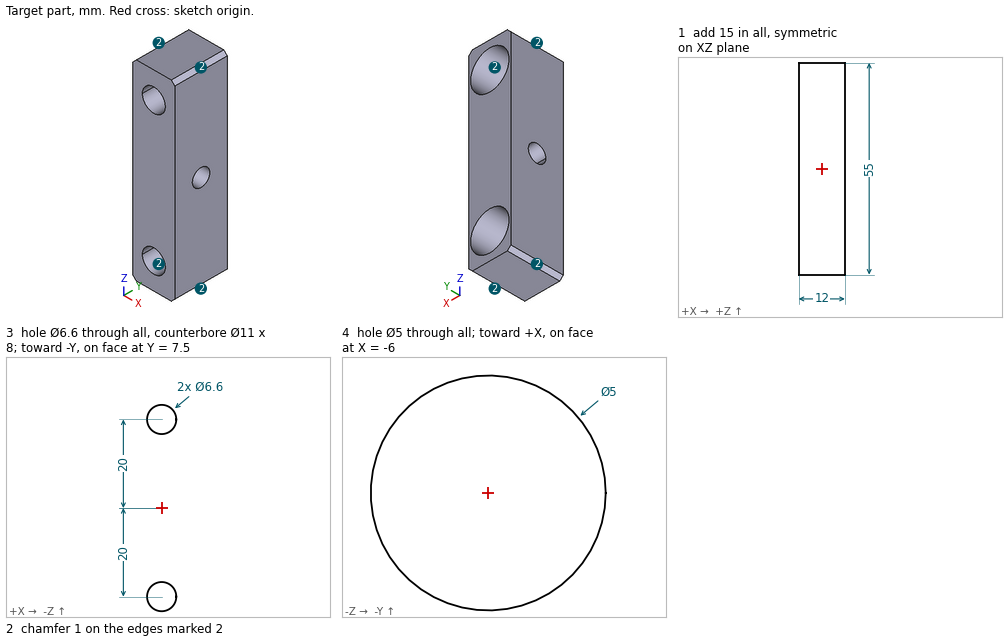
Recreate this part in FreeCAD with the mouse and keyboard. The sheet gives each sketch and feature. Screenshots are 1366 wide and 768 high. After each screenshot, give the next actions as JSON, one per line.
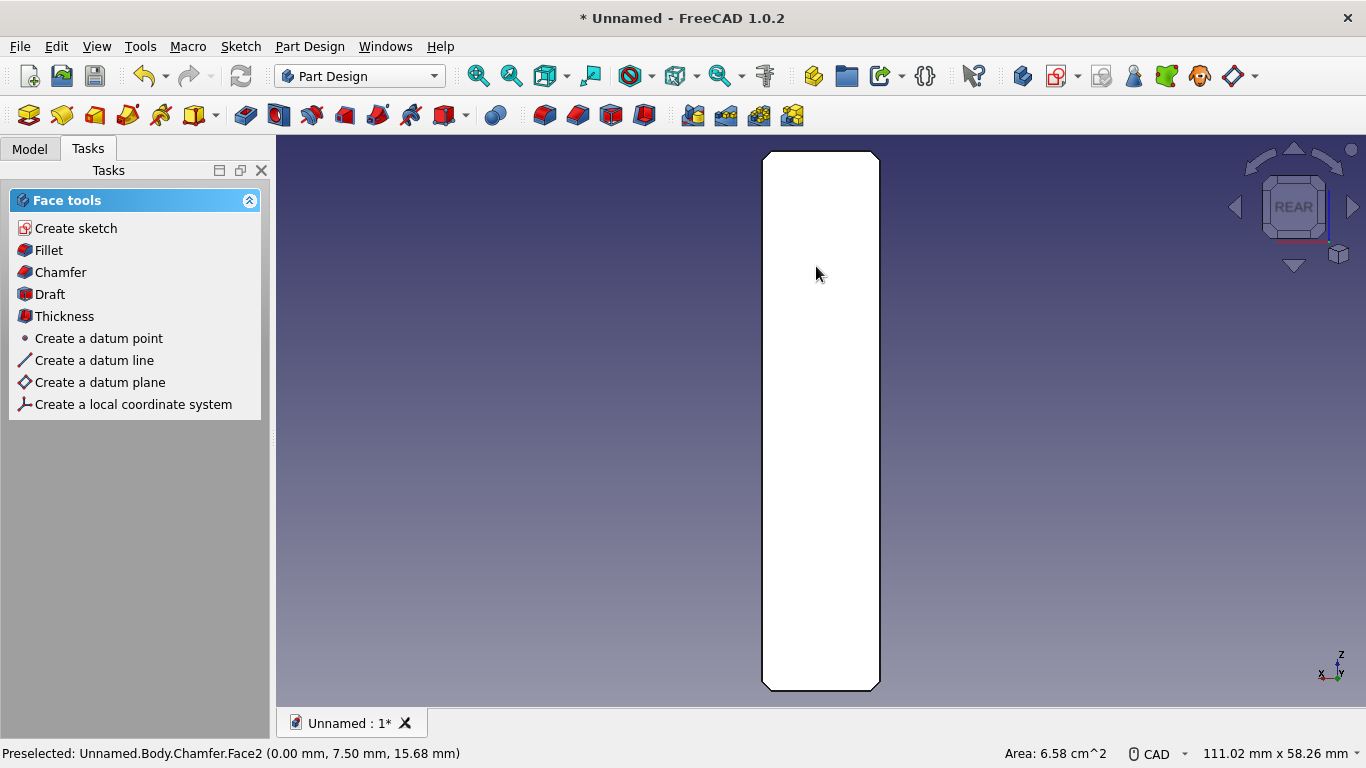
{"action": "left_click", "coordinate": [1056, 76]}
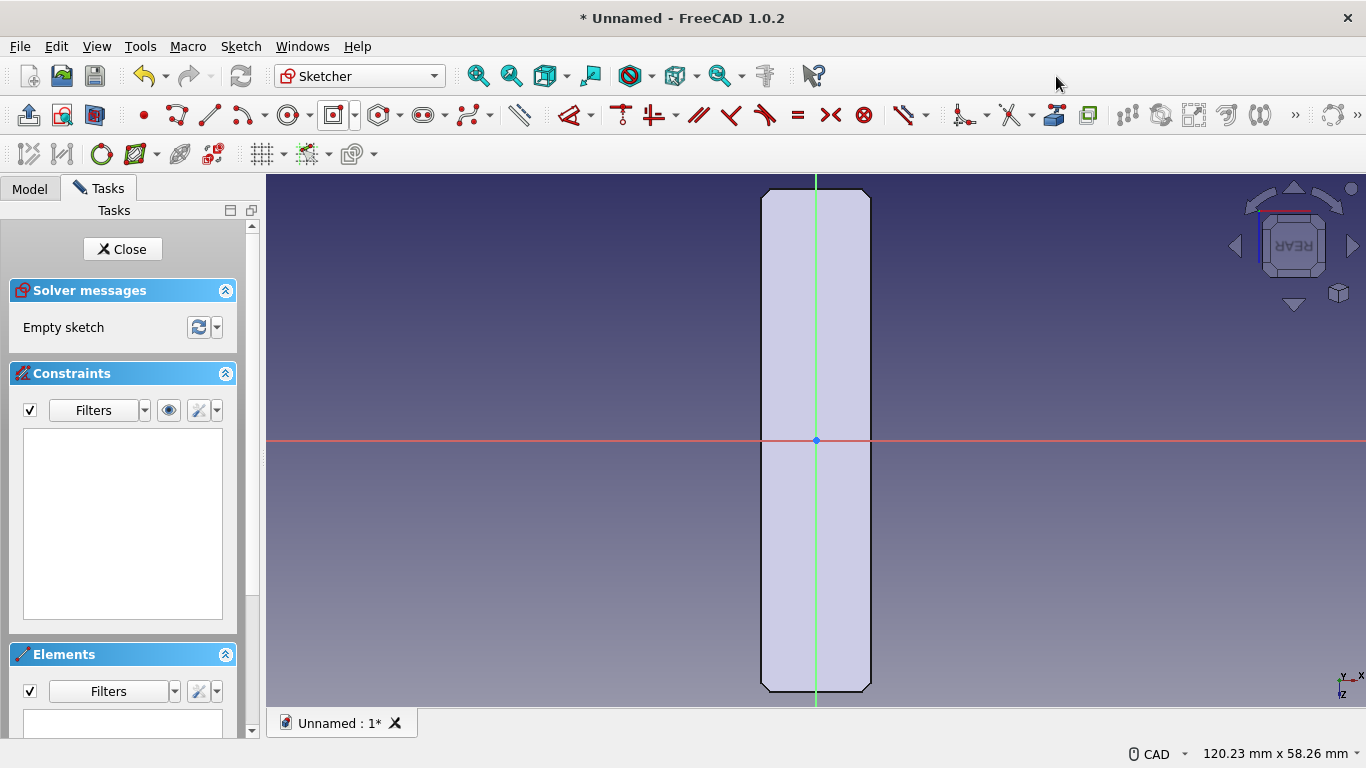
{"action": "left_click", "coordinate": [288, 116]}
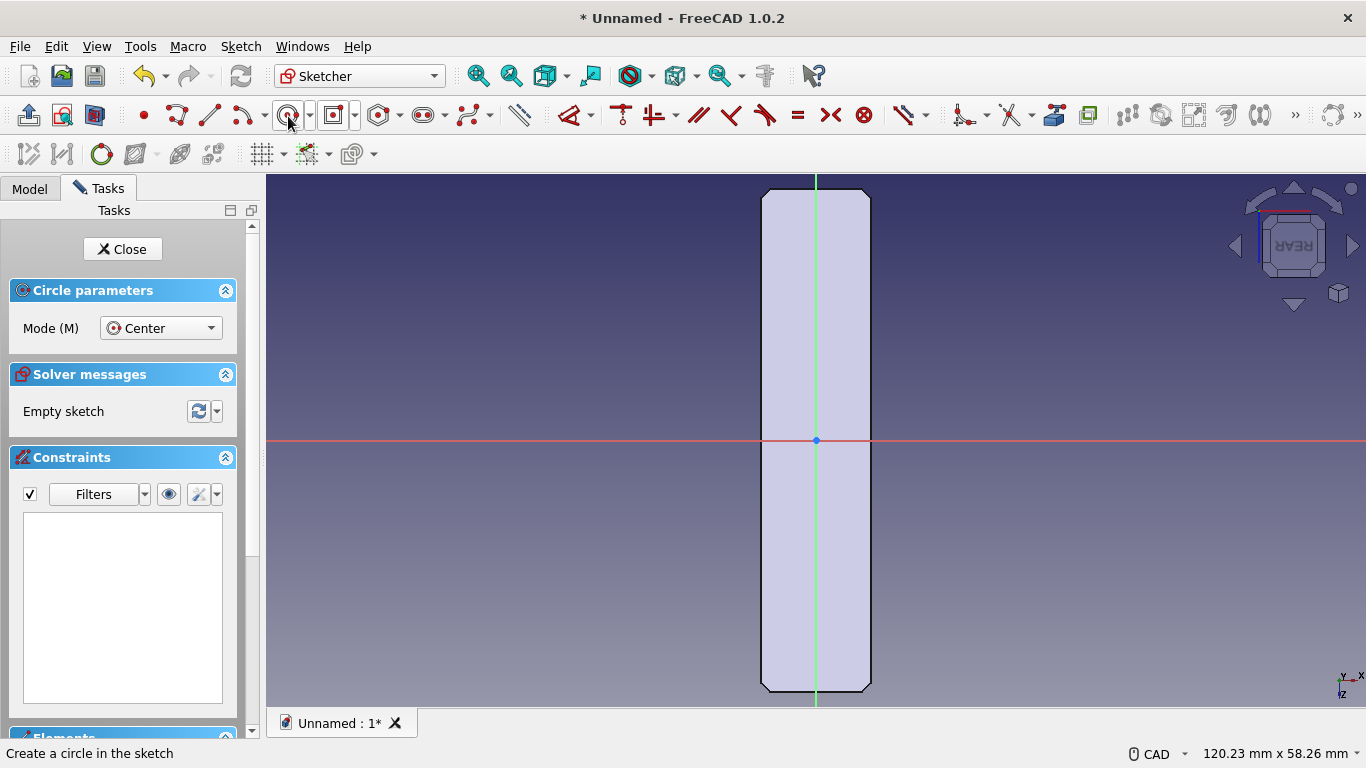
{"action": "left_click", "coordinate": [816, 258]}
{"action": "mouse_move", "coordinate": [837, 236]}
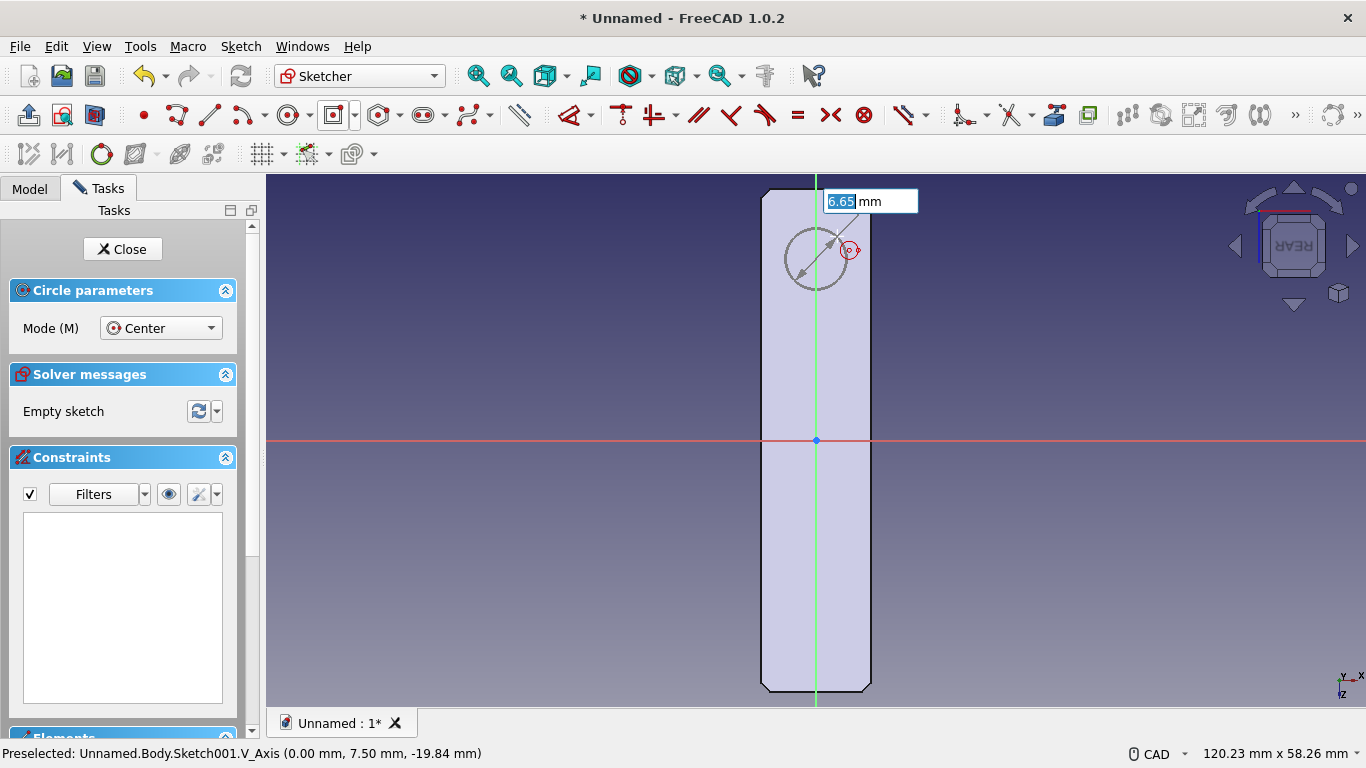
{"action": "type", "text": "6.6"}
{"action": "key", "text": "Return"}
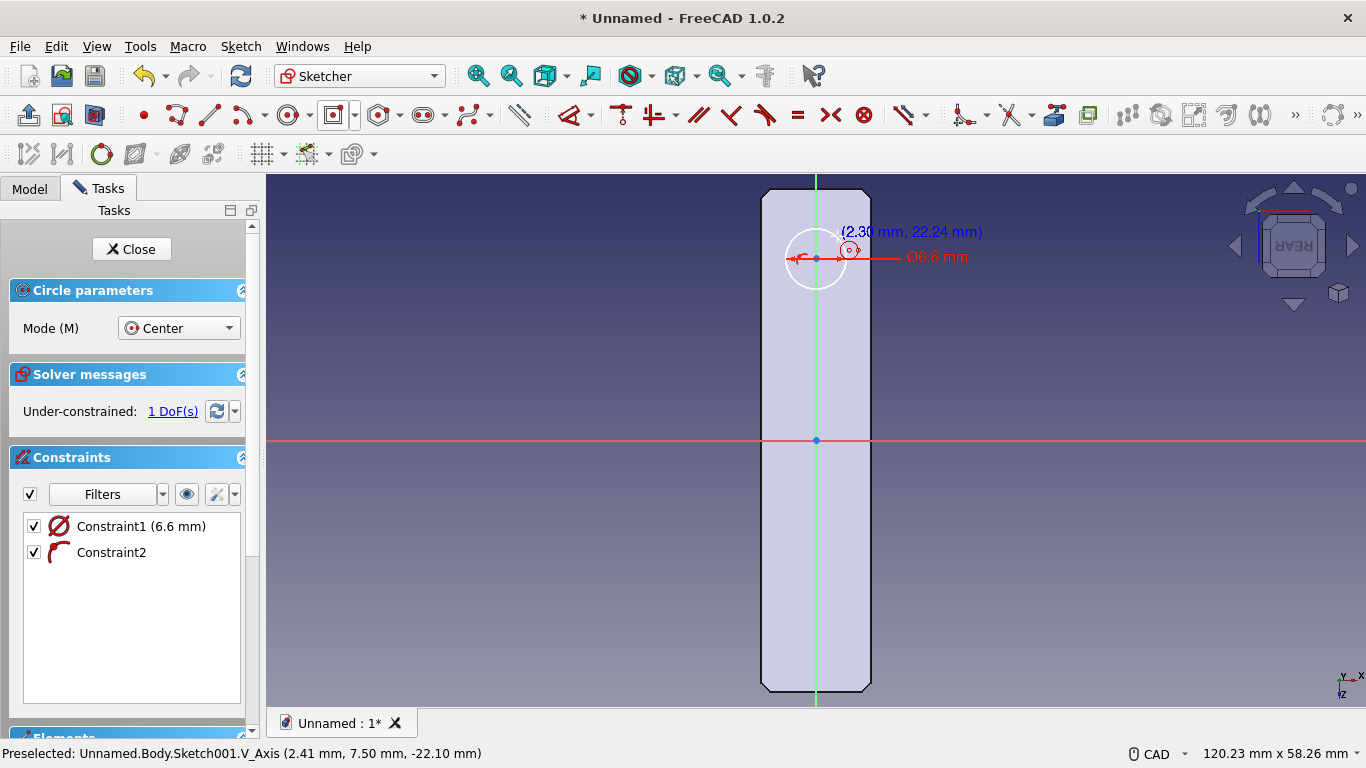
{"action": "left_click", "coordinate": [816, 623]}
{"action": "mouse_move", "coordinate": [837, 602]}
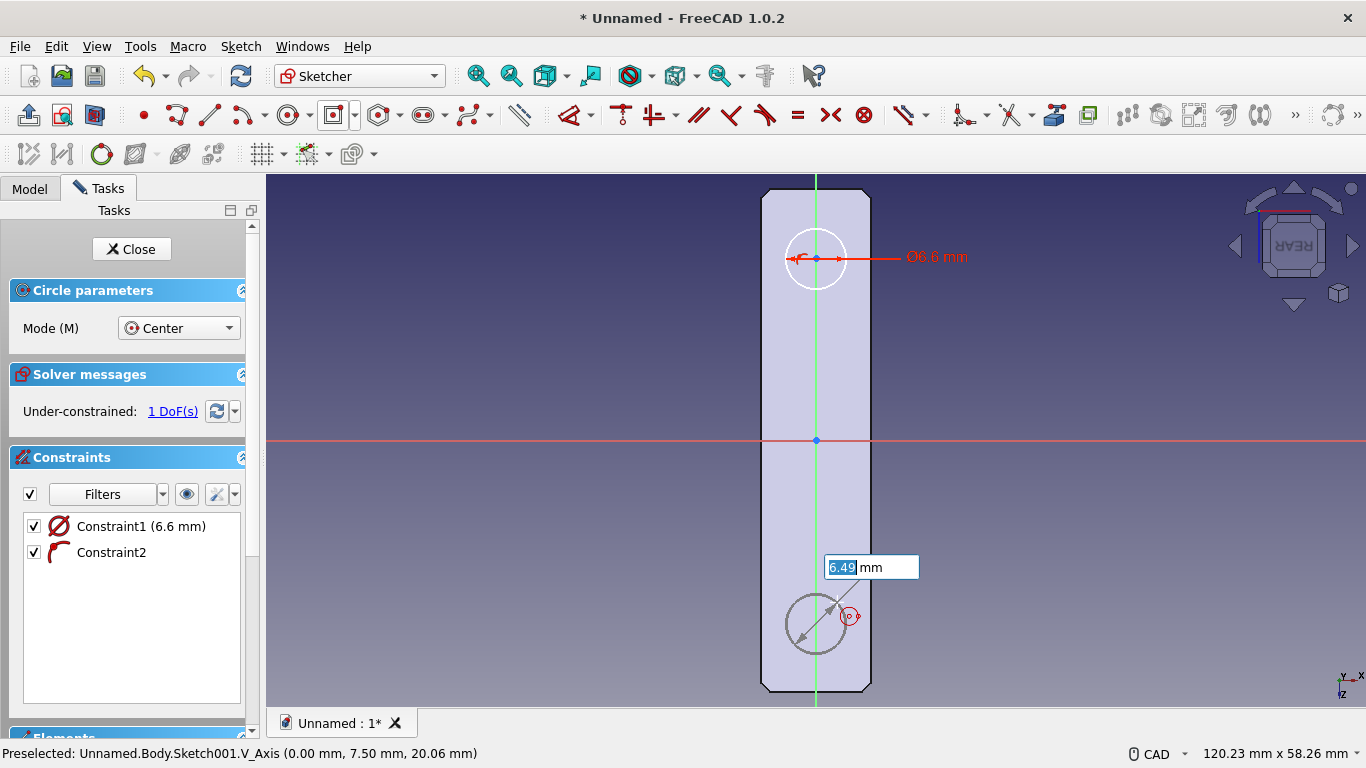
{"action": "type", "text": "6.6"}
{"action": "key", "text": "Return"}
{"action": "key", "text": "Escape"}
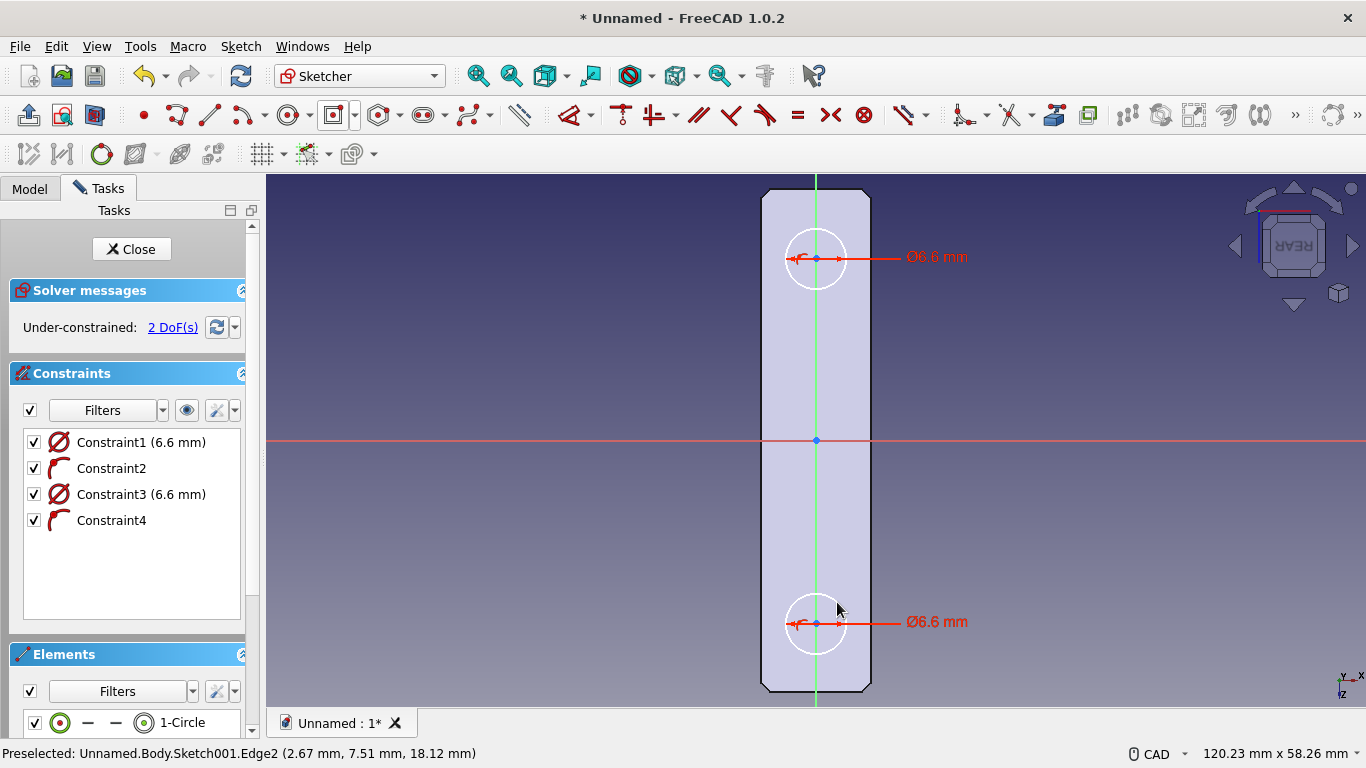
{"action": "left_click", "coordinate": [816, 259]}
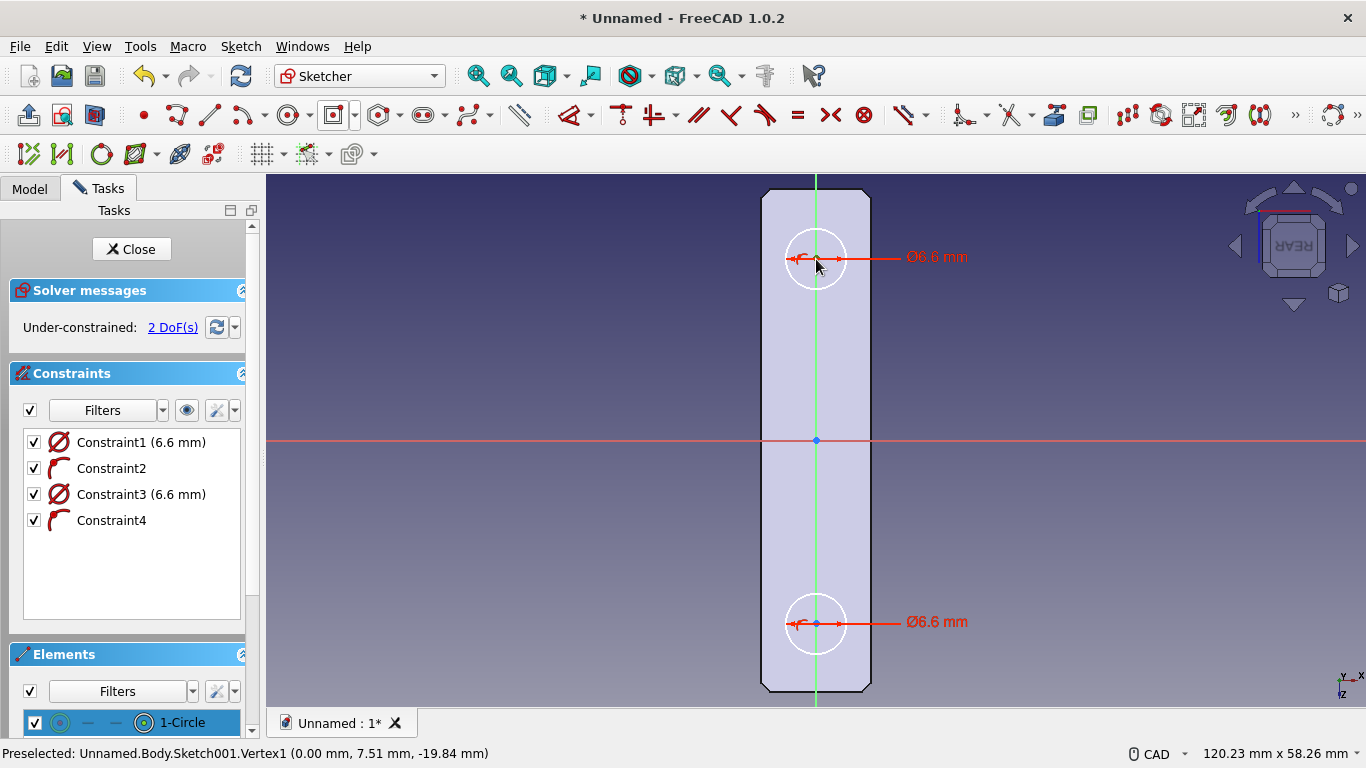
{"action": "left_click", "coordinate": [590, 116]}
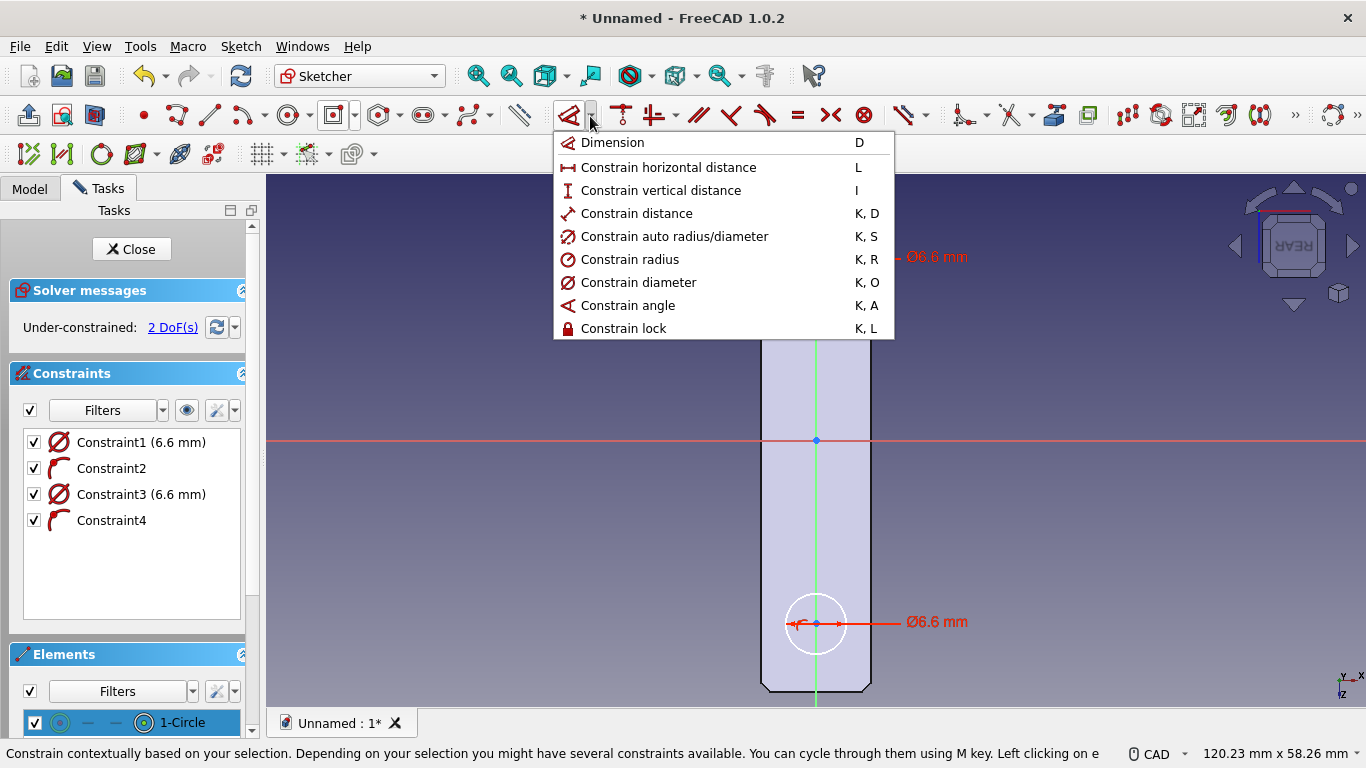
{"action": "left_click", "coordinate": [724, 190]}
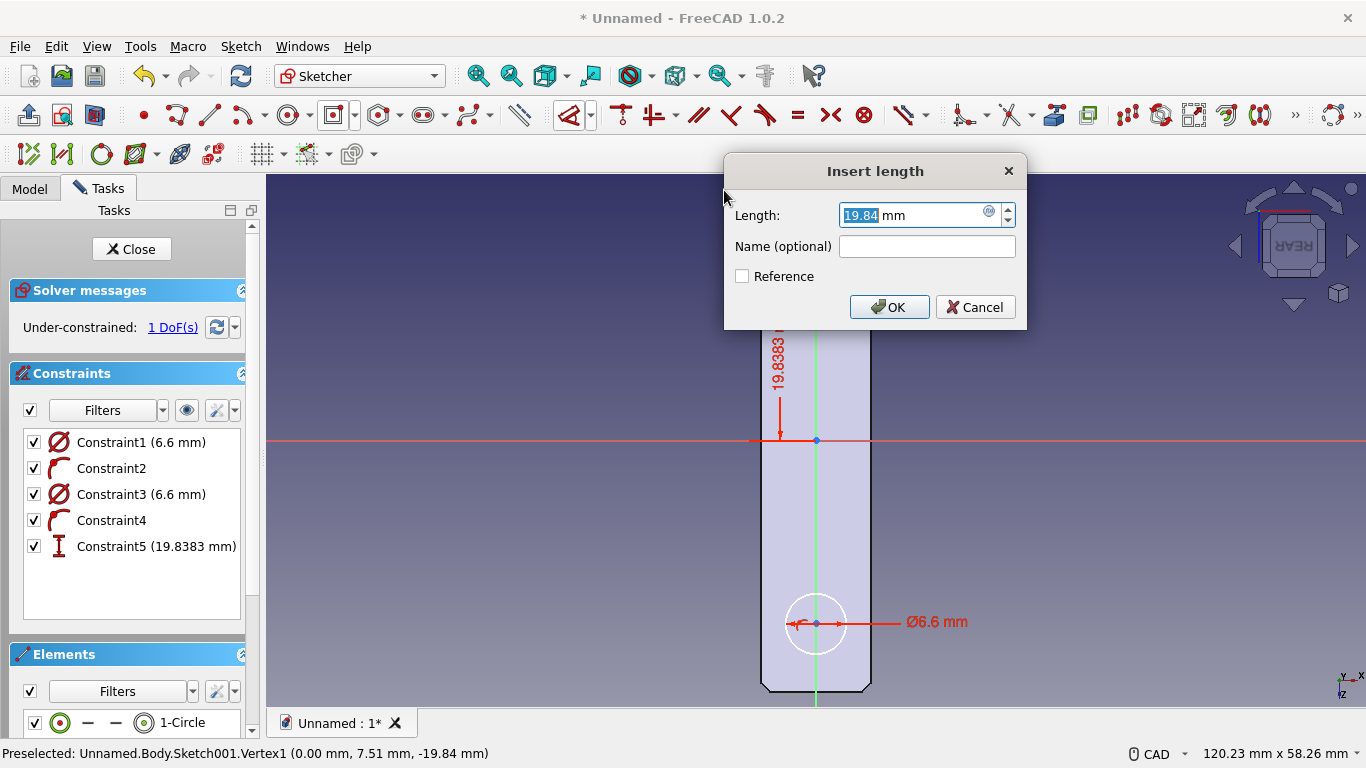
{"action": "type", "text": "20"}
{"action": "key", "text": "Return"}